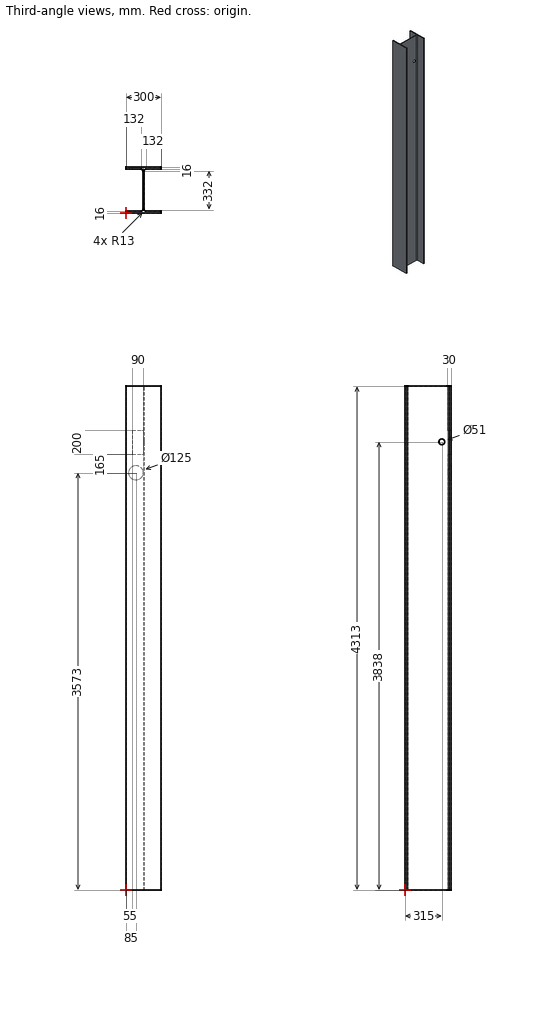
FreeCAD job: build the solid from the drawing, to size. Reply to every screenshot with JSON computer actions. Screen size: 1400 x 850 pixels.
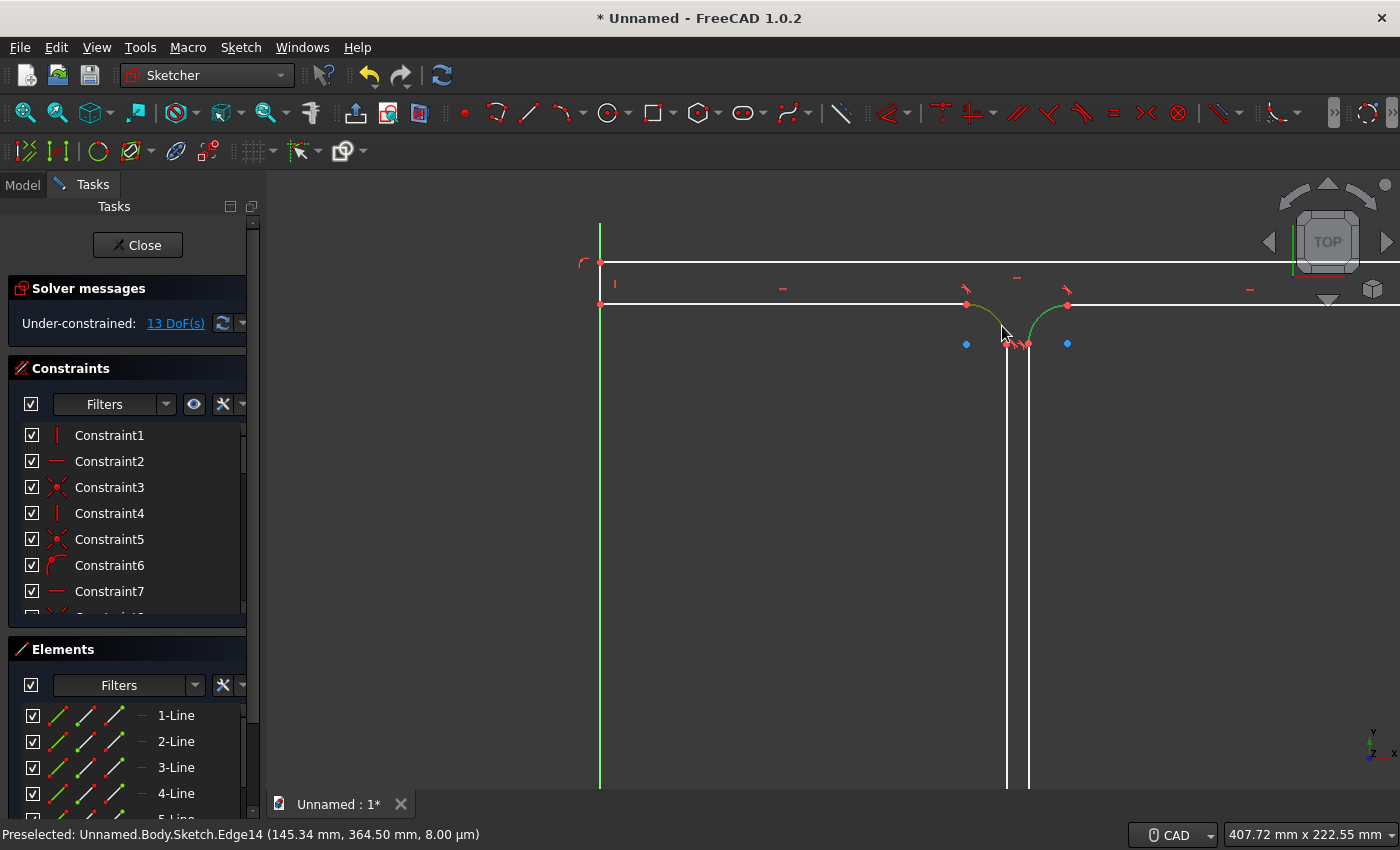
{"action": "scroll", "coordinate": [617, 292], "scroll_direction": "down", "scroll_amount": 5}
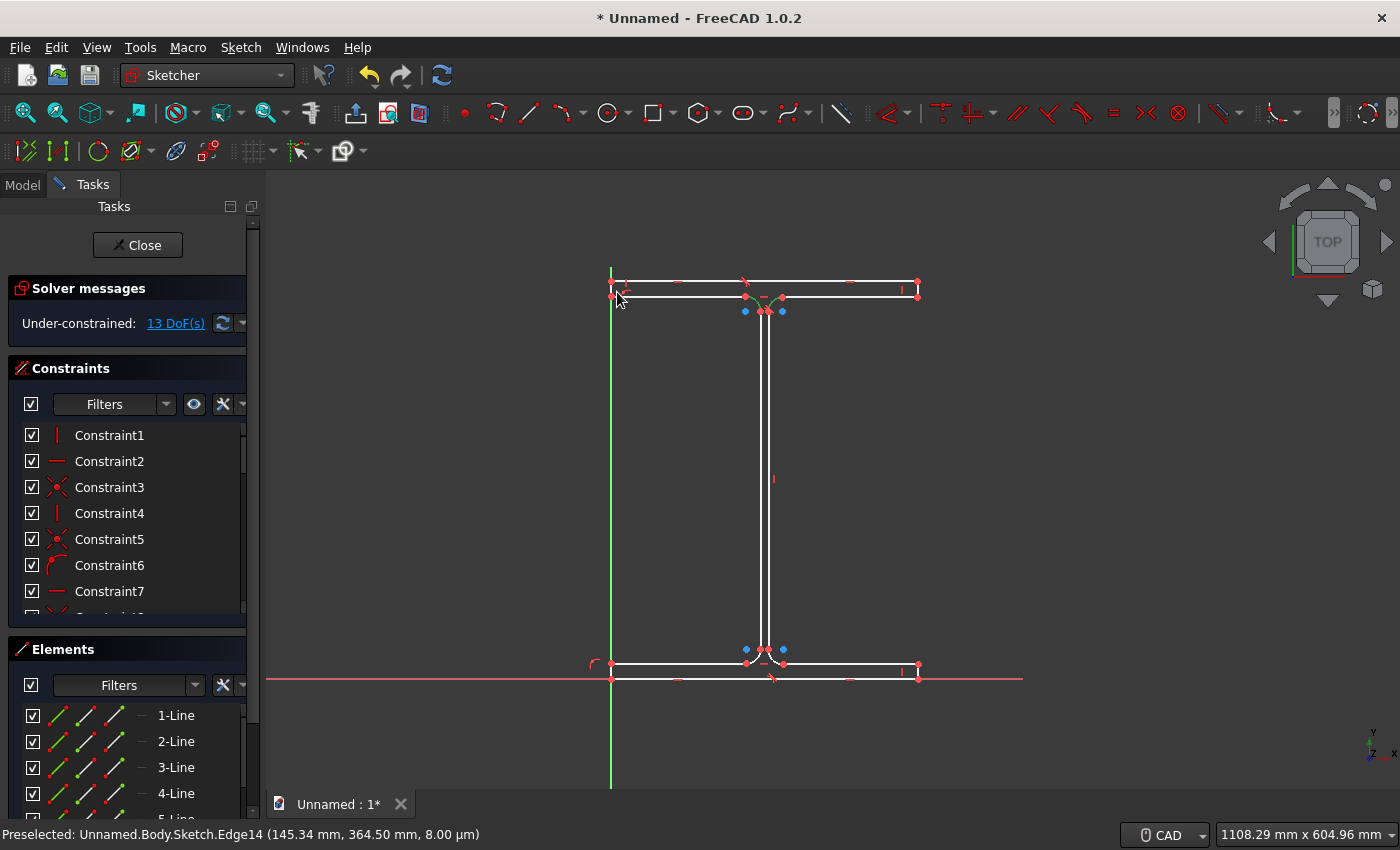
{"action": "scroll", "coordinate": [753, 662], "scroll_direction": "up", "scroll_amount": 4}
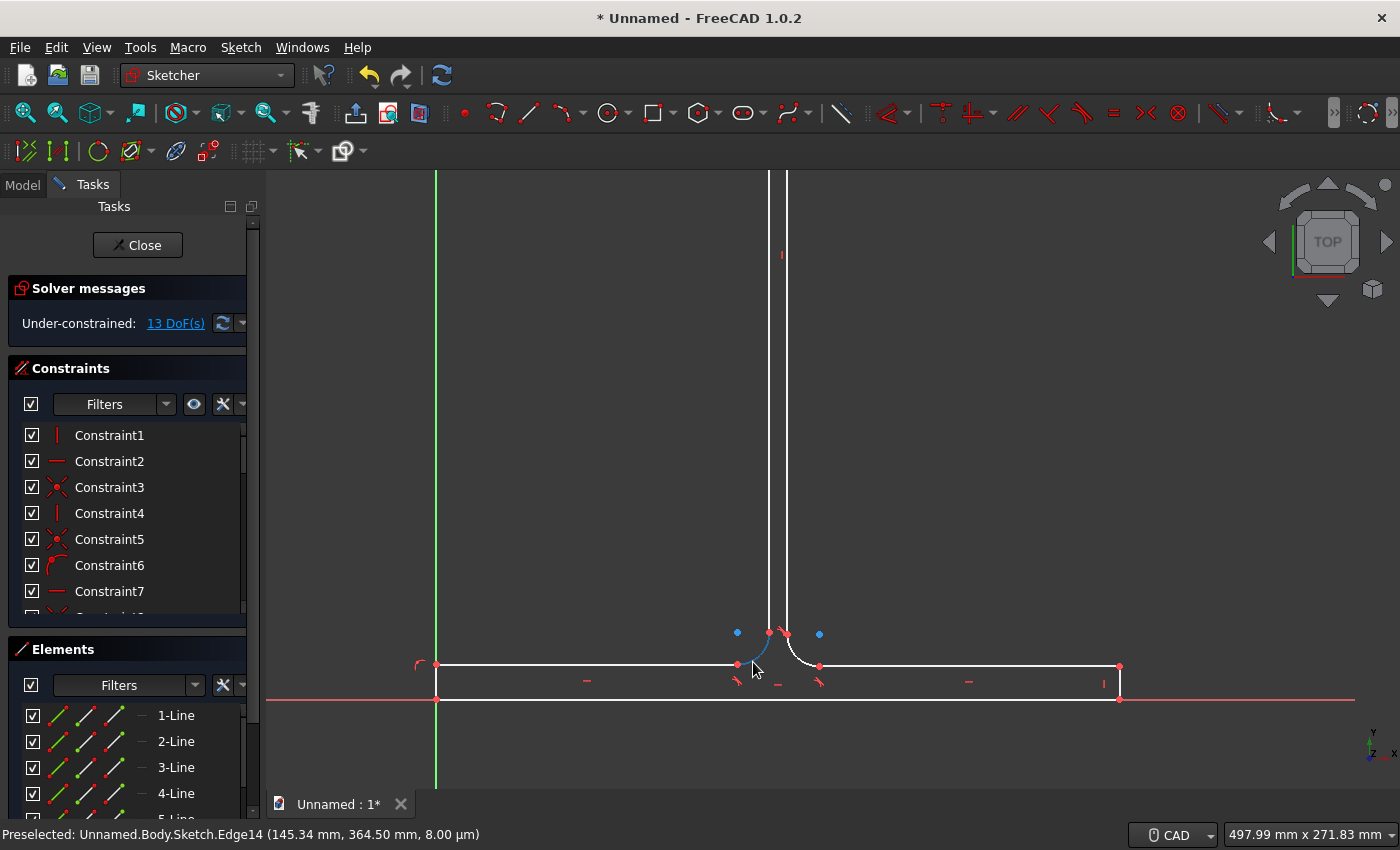
{"action": "left_click", "coordinate": [752, 661]}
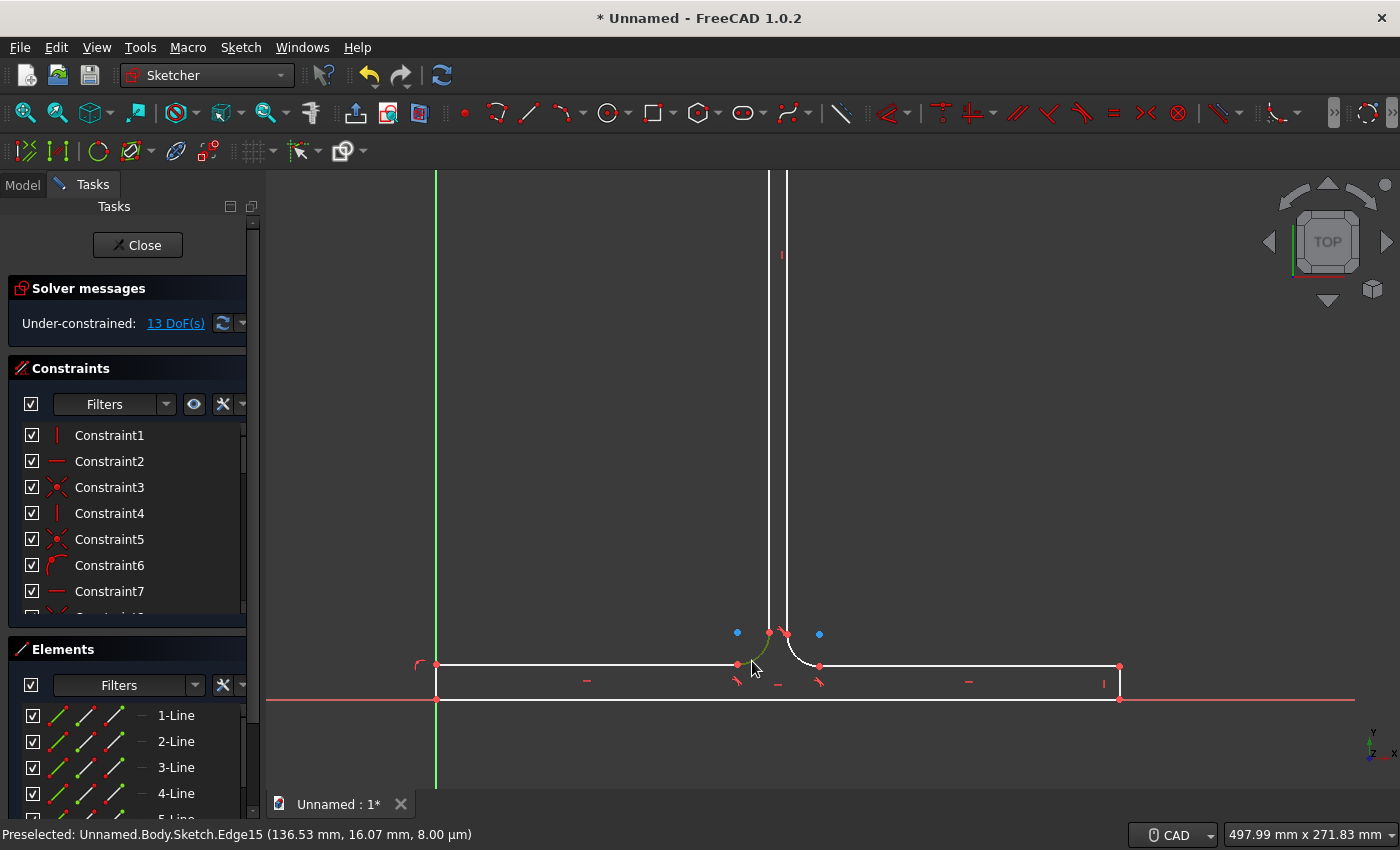
{"action": "left_click", "coordinate": [791, 649]}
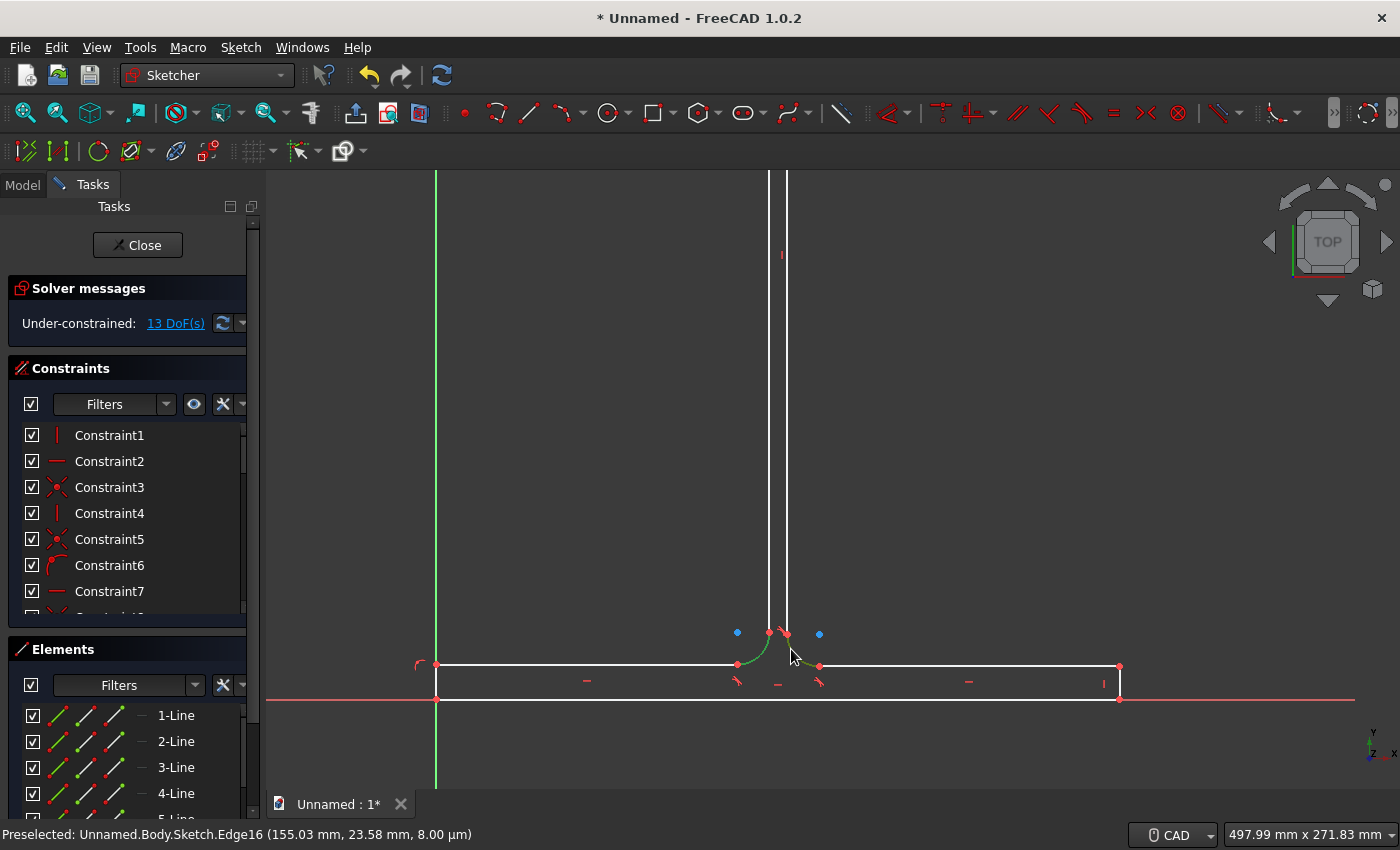
{"action": "left_click", "coordinate": [1114, 114]}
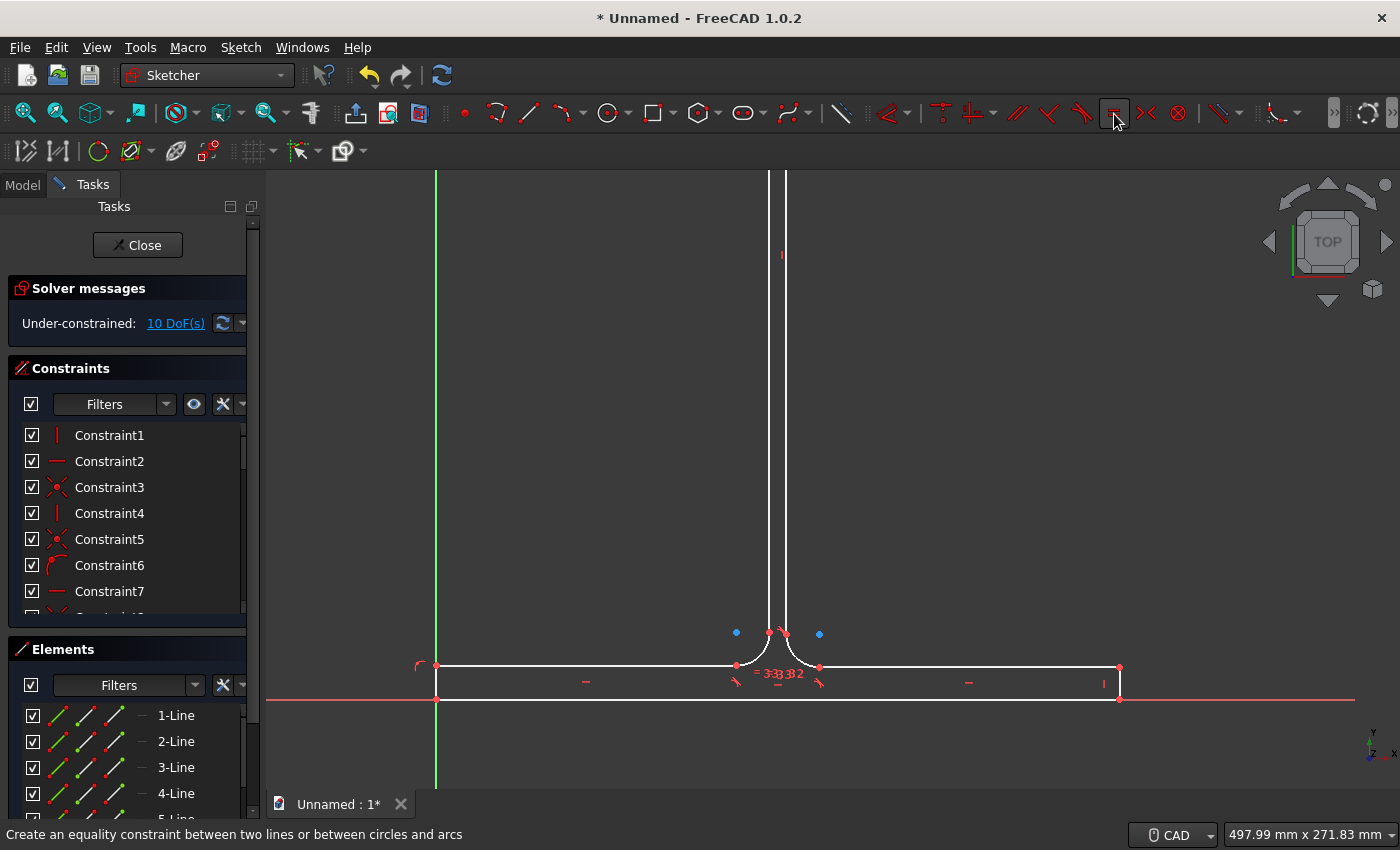
{"action": "scroll", "coordinate": [753, 662], "scroll_direction": "down", "scroll_amount": 4}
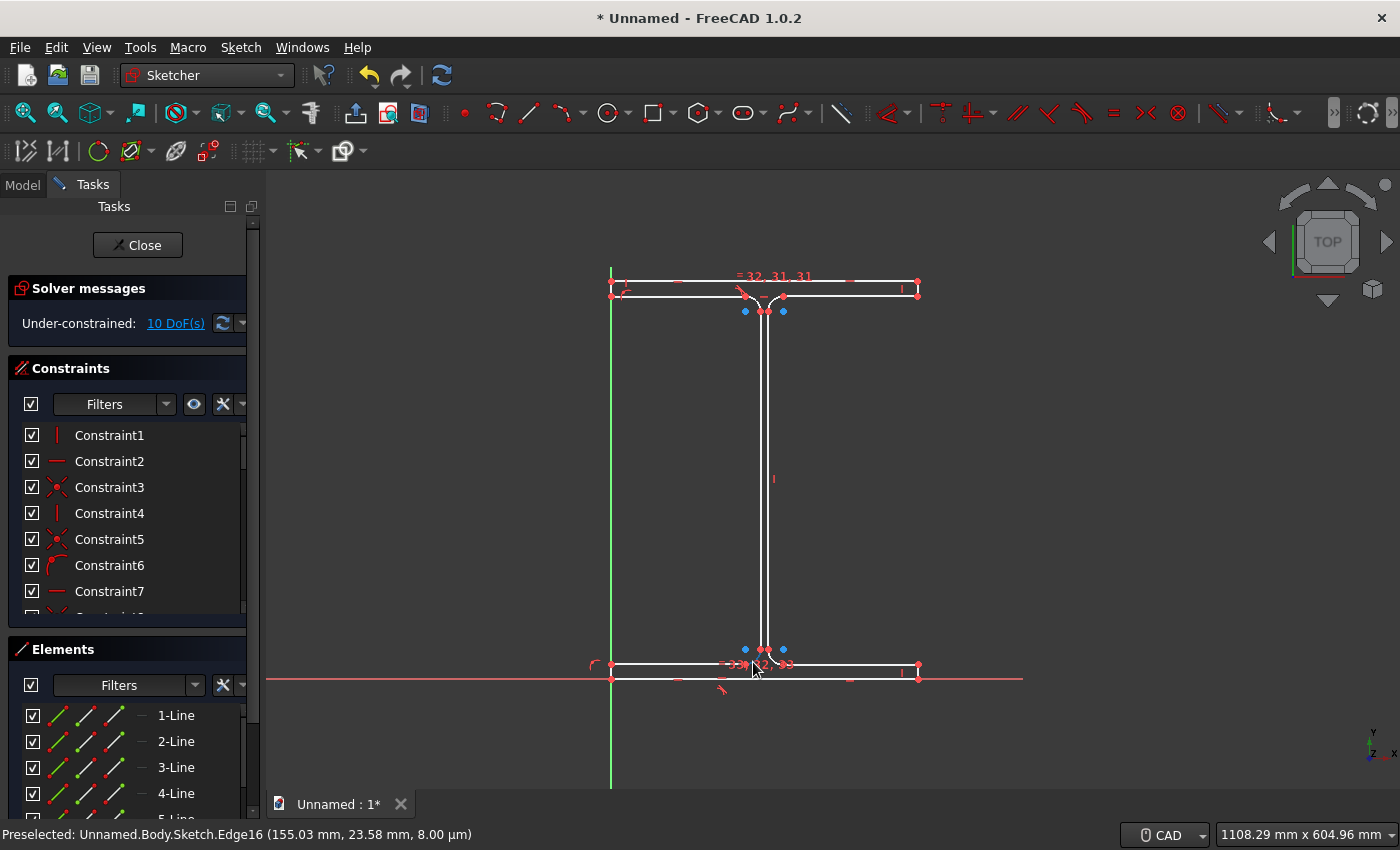
{"action": "scroll", "coordinate": [776, 298], "scroll_direction": "up", "scroll_amount": 6}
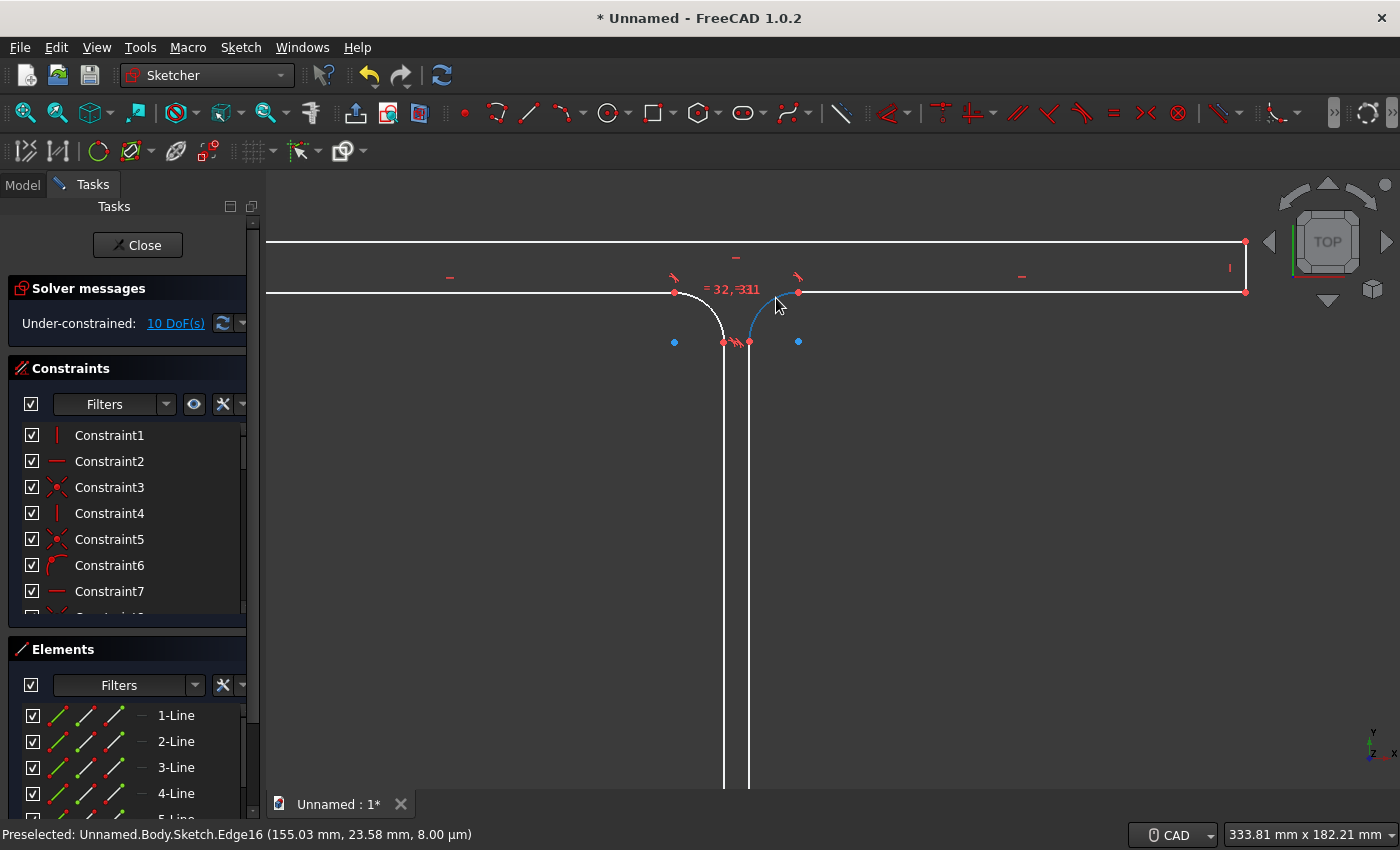
{"action": "left_click", "coordinate": [776, 298]}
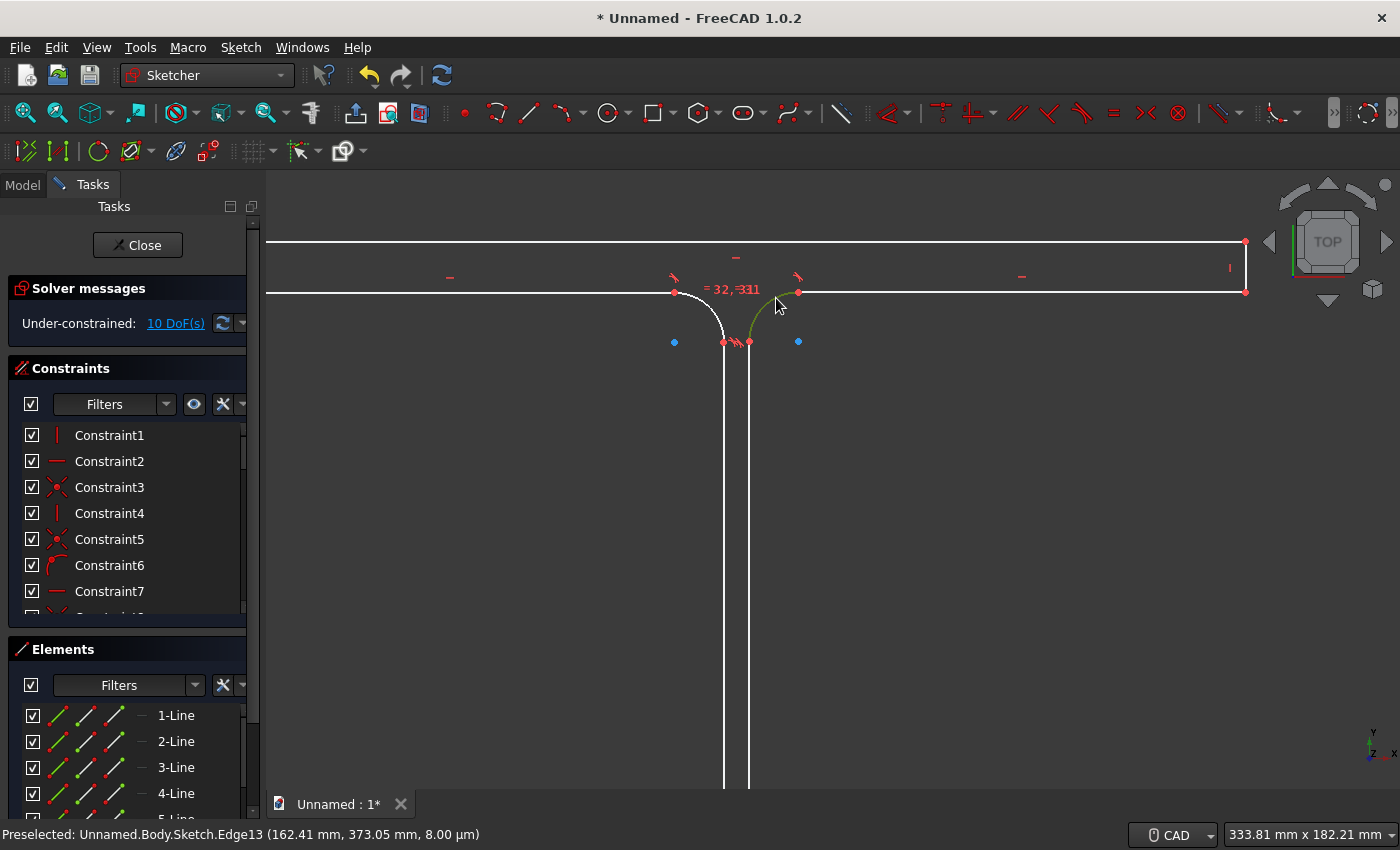
{"action": "key", "text": "k r"}